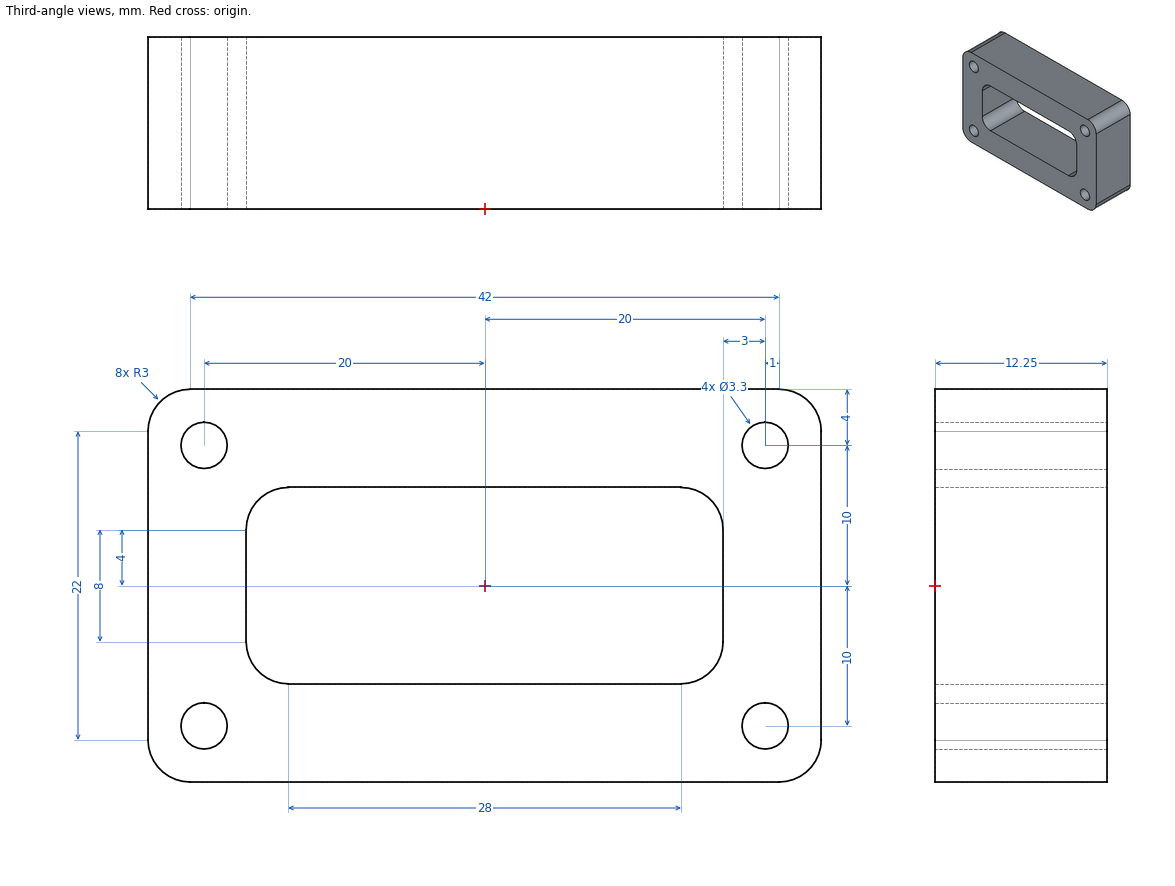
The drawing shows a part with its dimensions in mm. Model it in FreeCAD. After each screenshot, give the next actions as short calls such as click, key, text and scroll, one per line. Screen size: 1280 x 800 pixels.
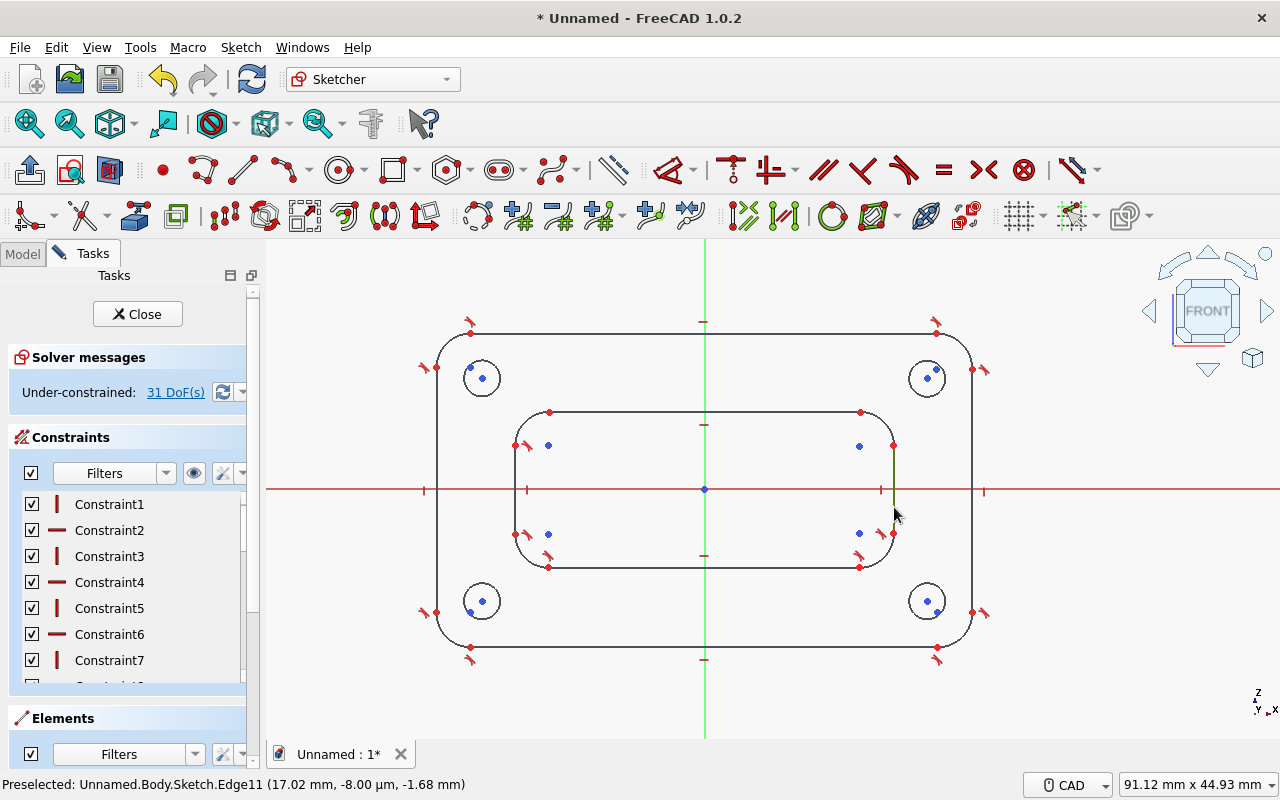
click(890, 431)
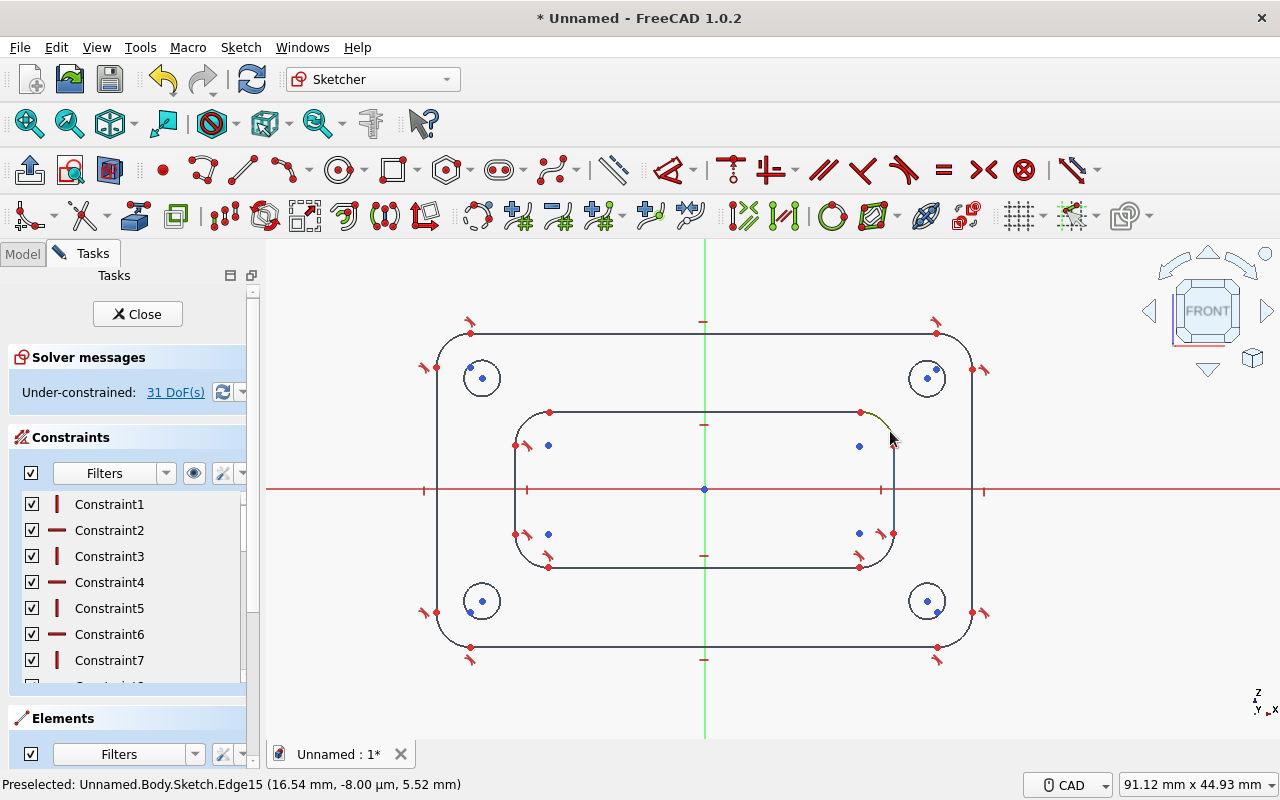
click(904, 170)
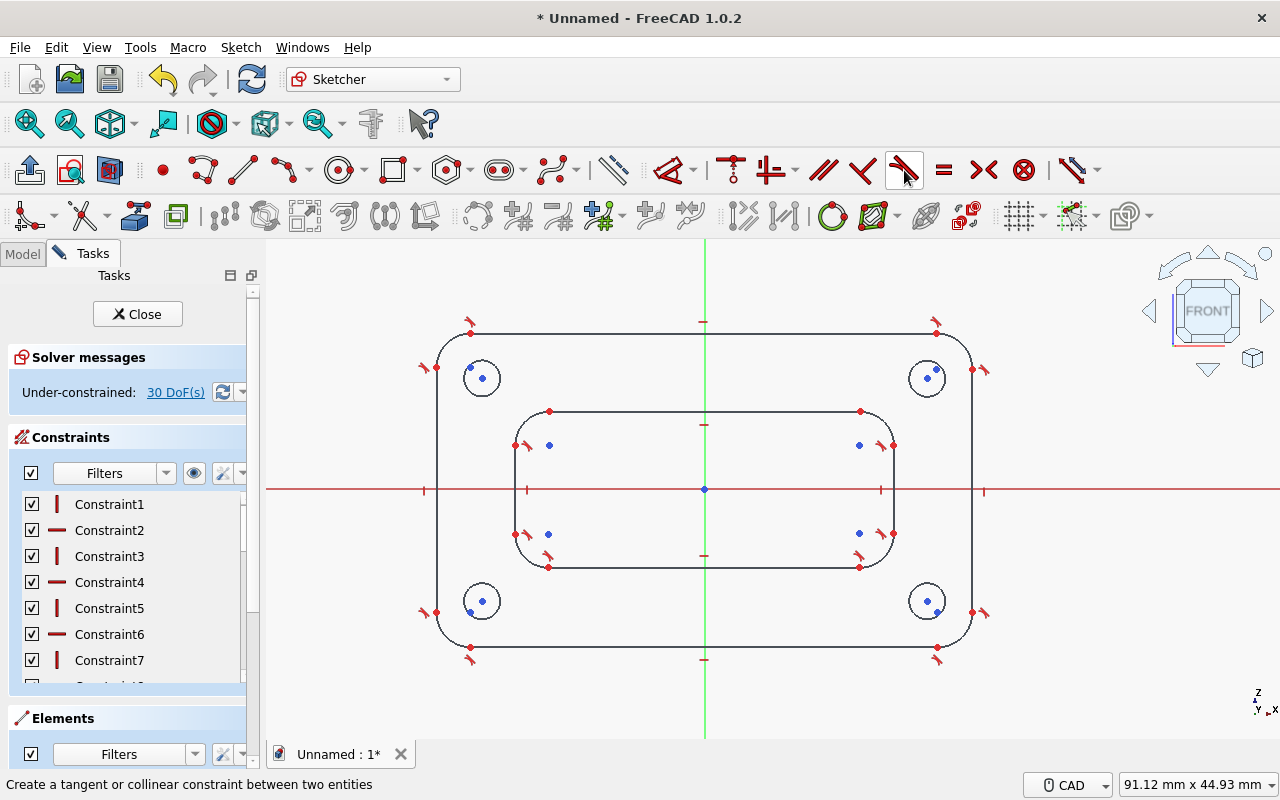
click(767, 412)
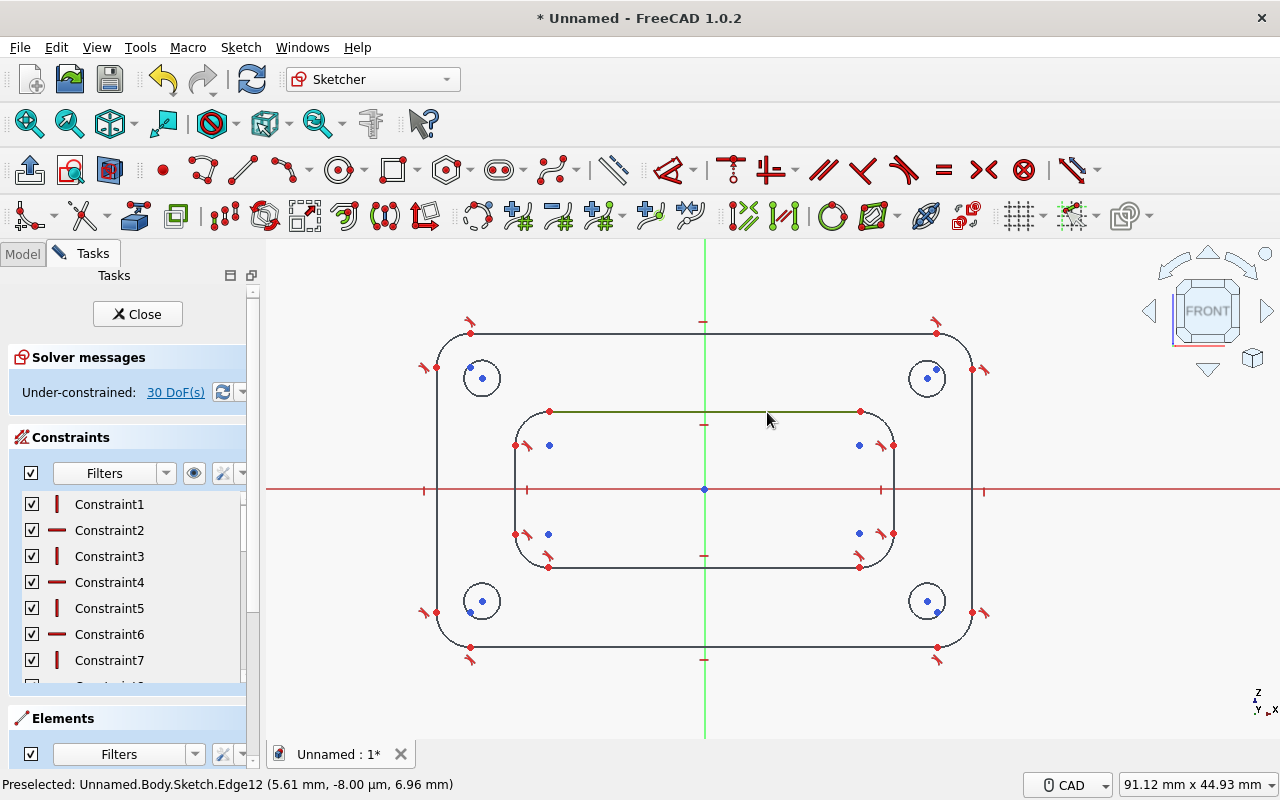
click(890, 431)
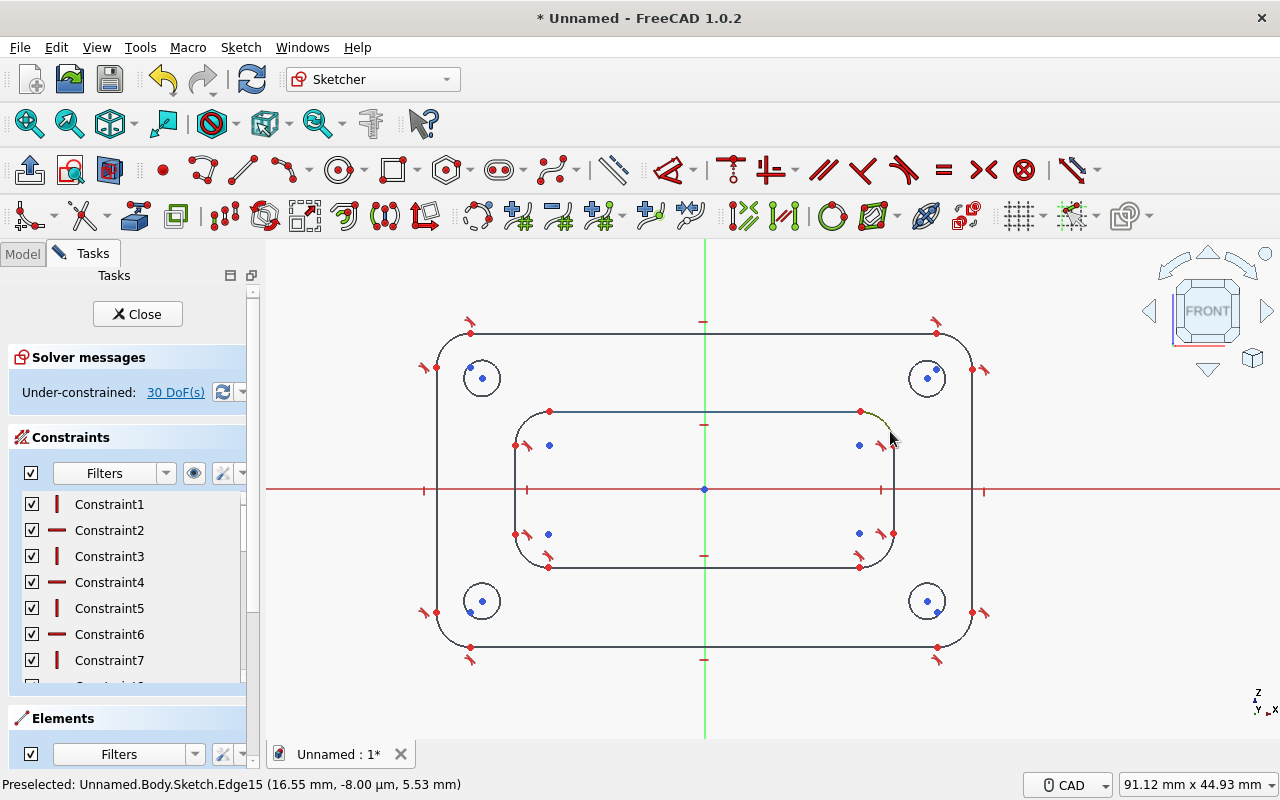
click(904, 170)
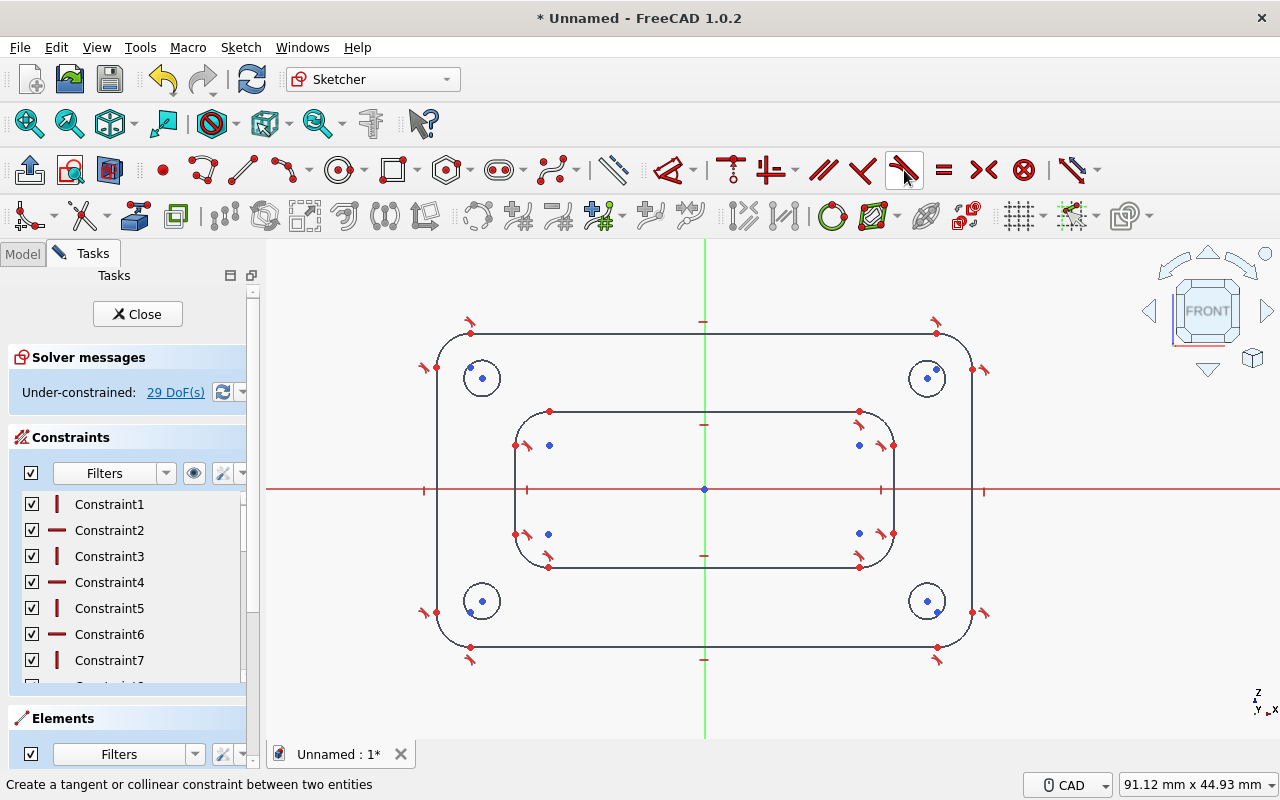
click(767, 412)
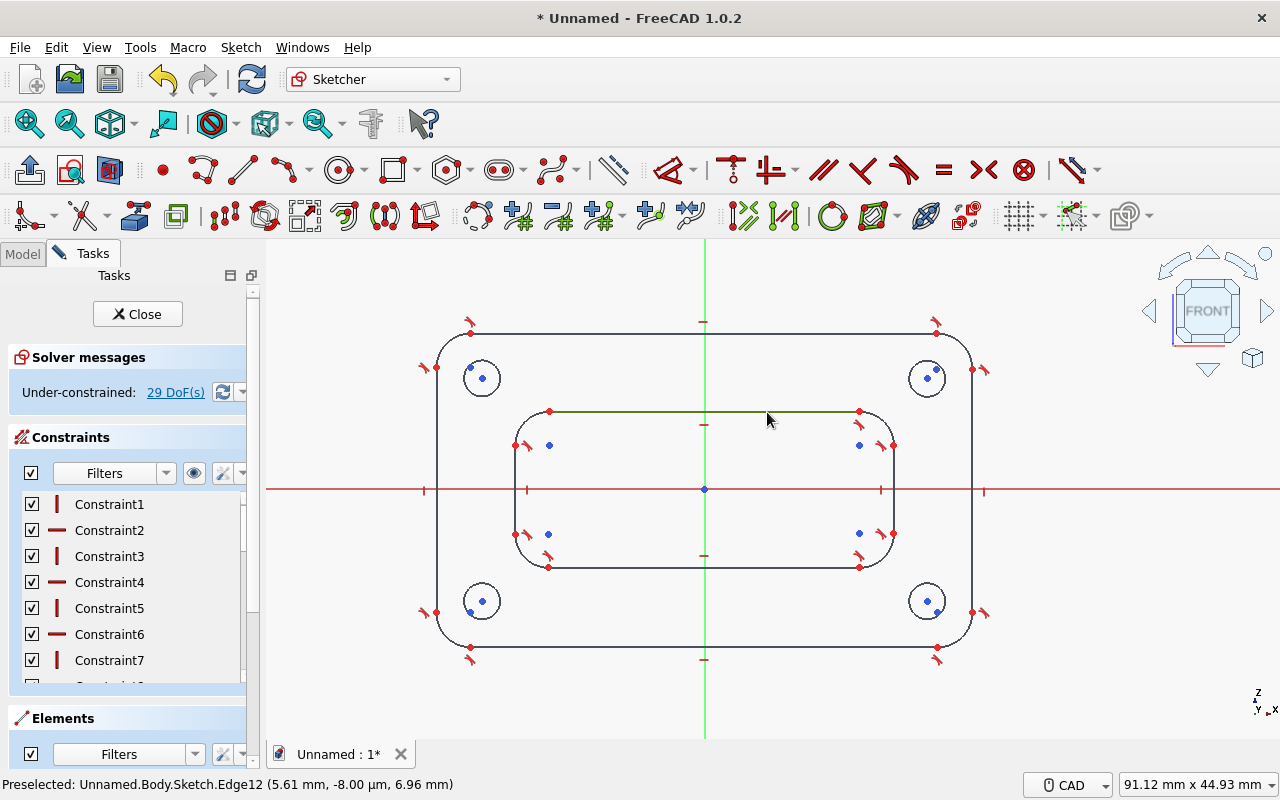
click(534, 416)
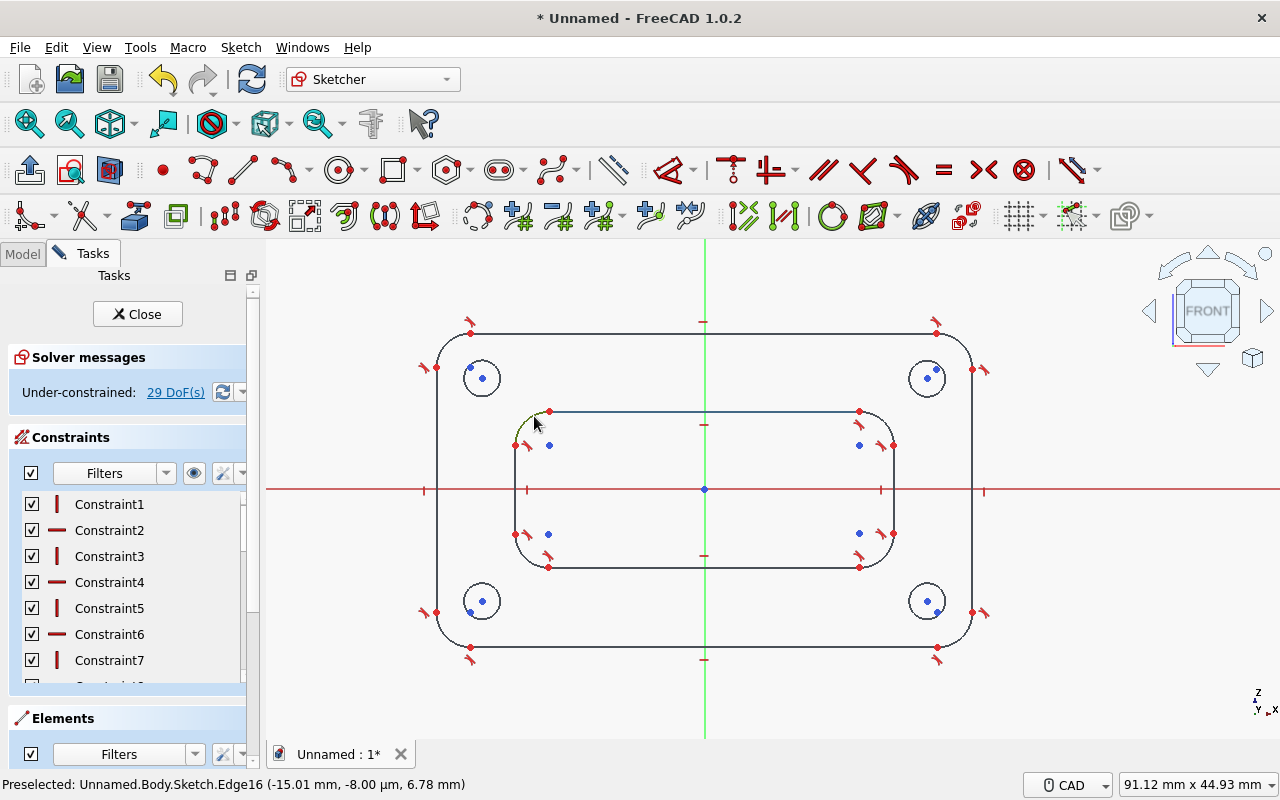
click(904, 170)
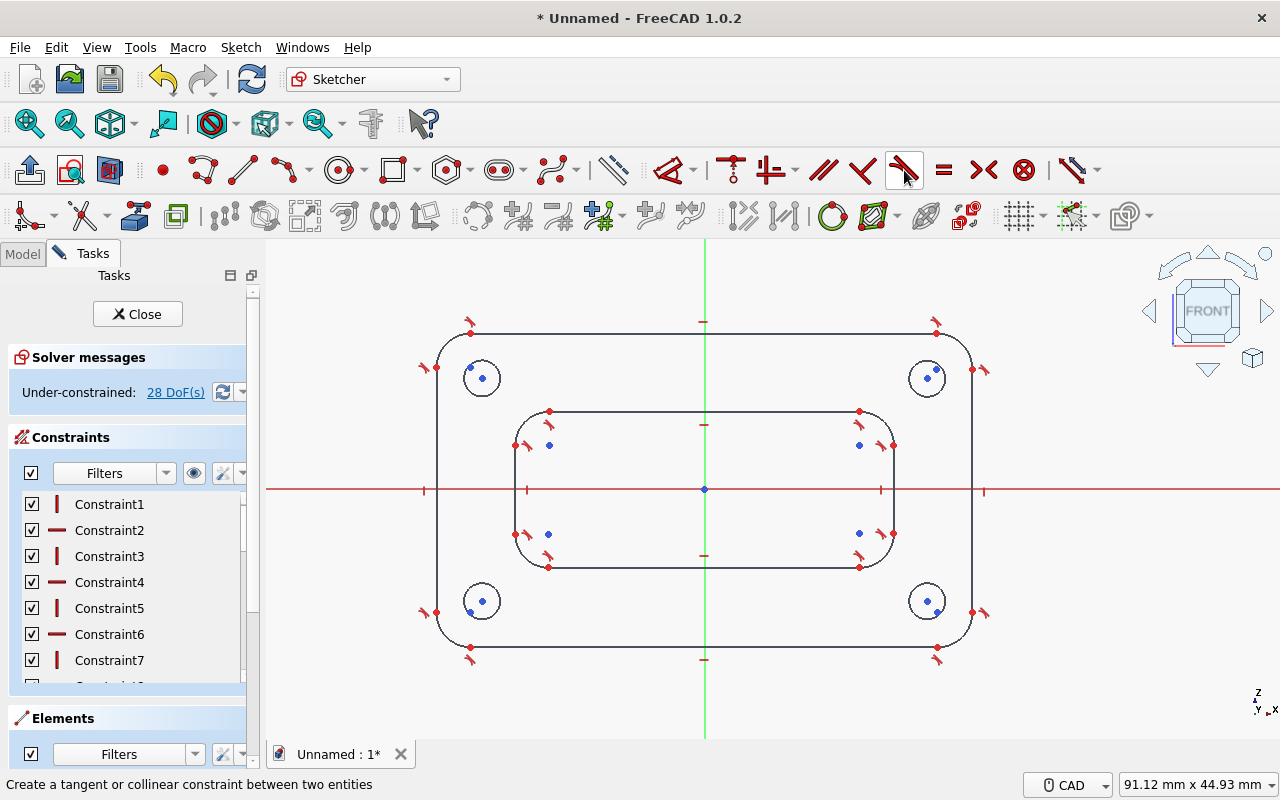
click(455, 337)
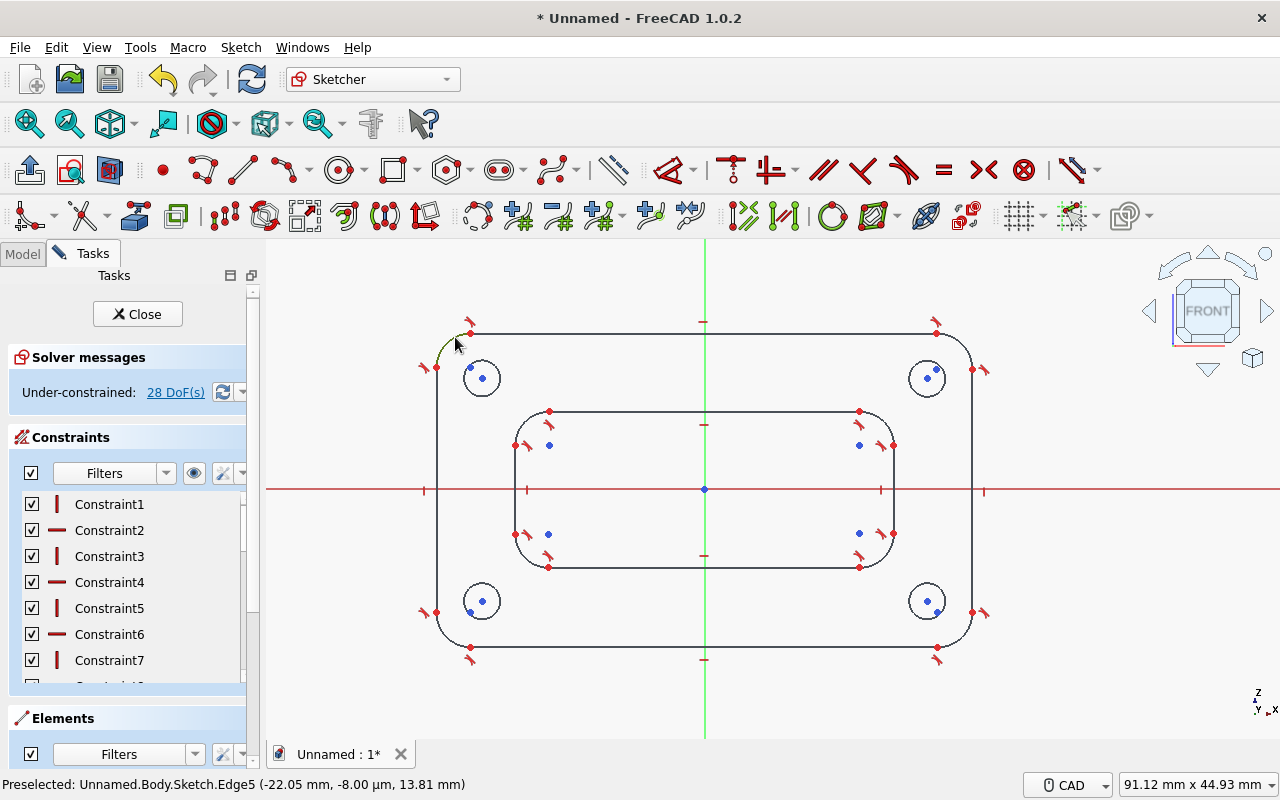
click(968, 353)